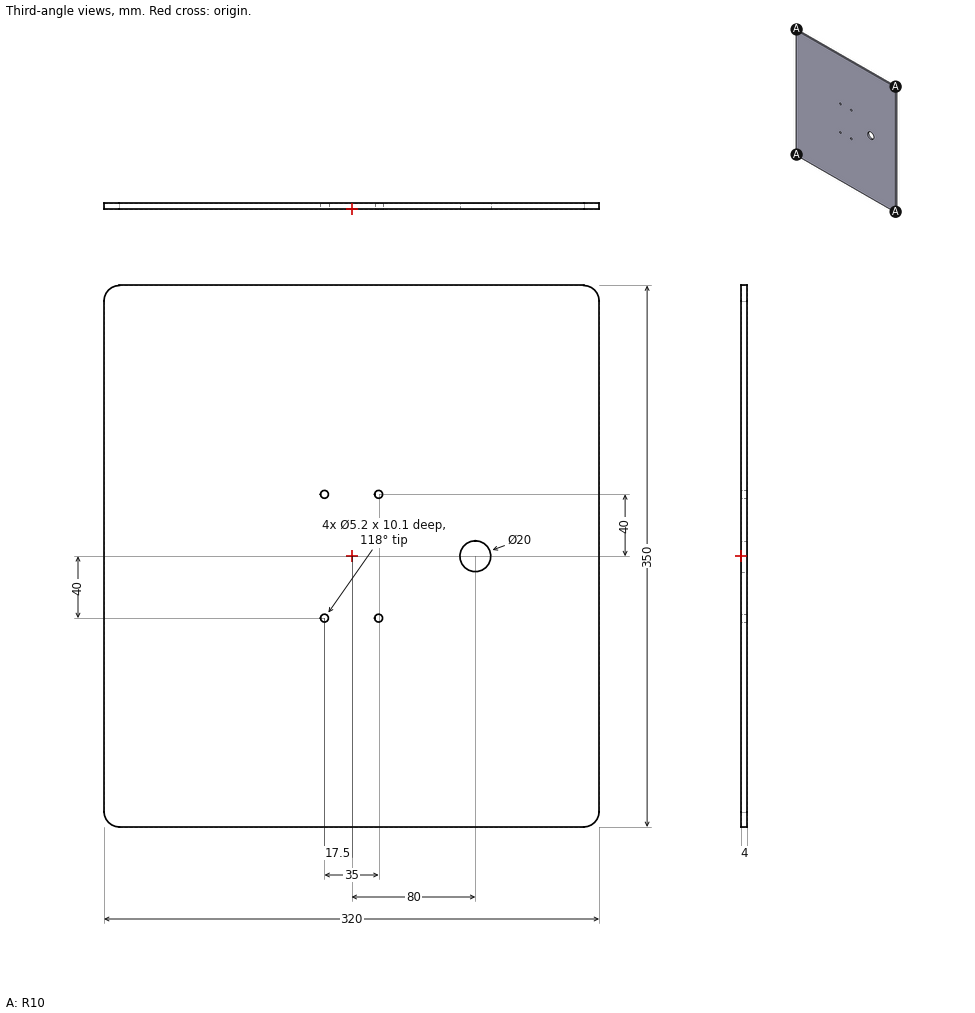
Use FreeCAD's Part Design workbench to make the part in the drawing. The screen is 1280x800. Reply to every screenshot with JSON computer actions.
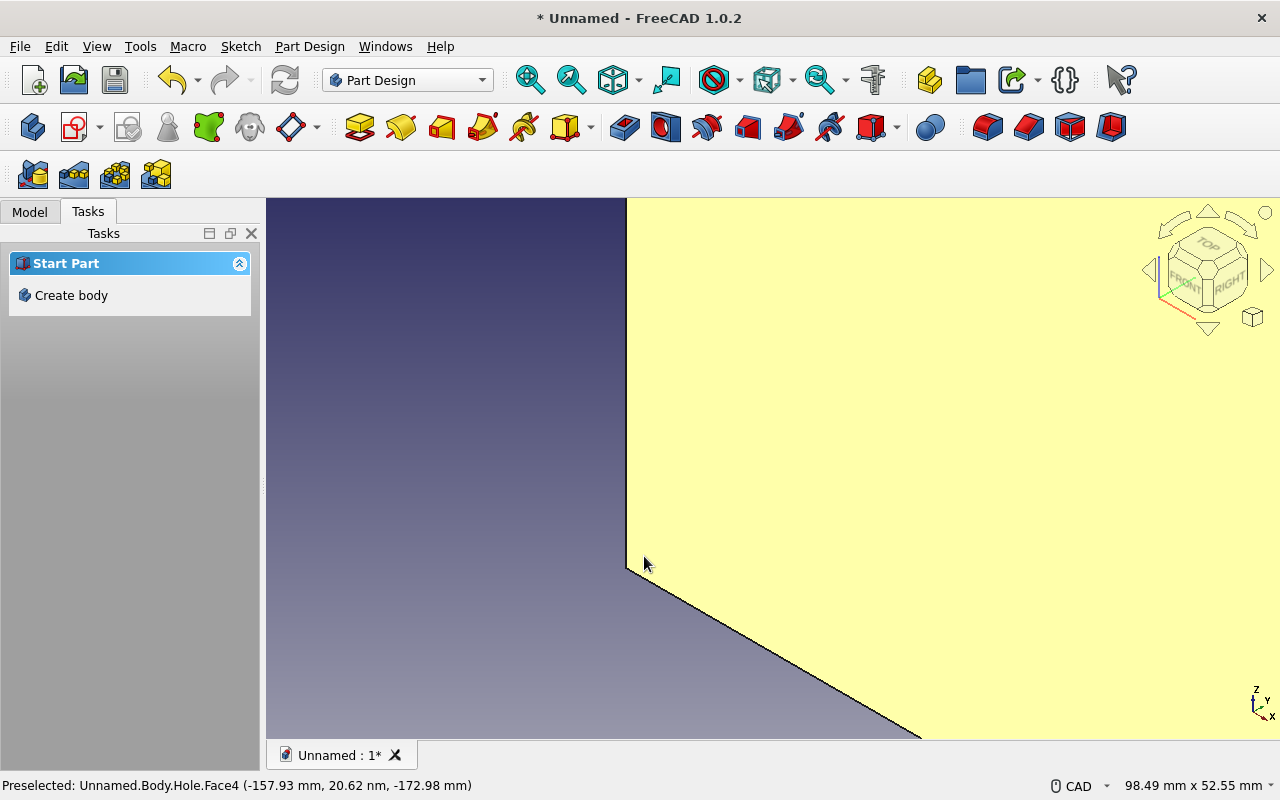
{"action": "key", "text": "v f"}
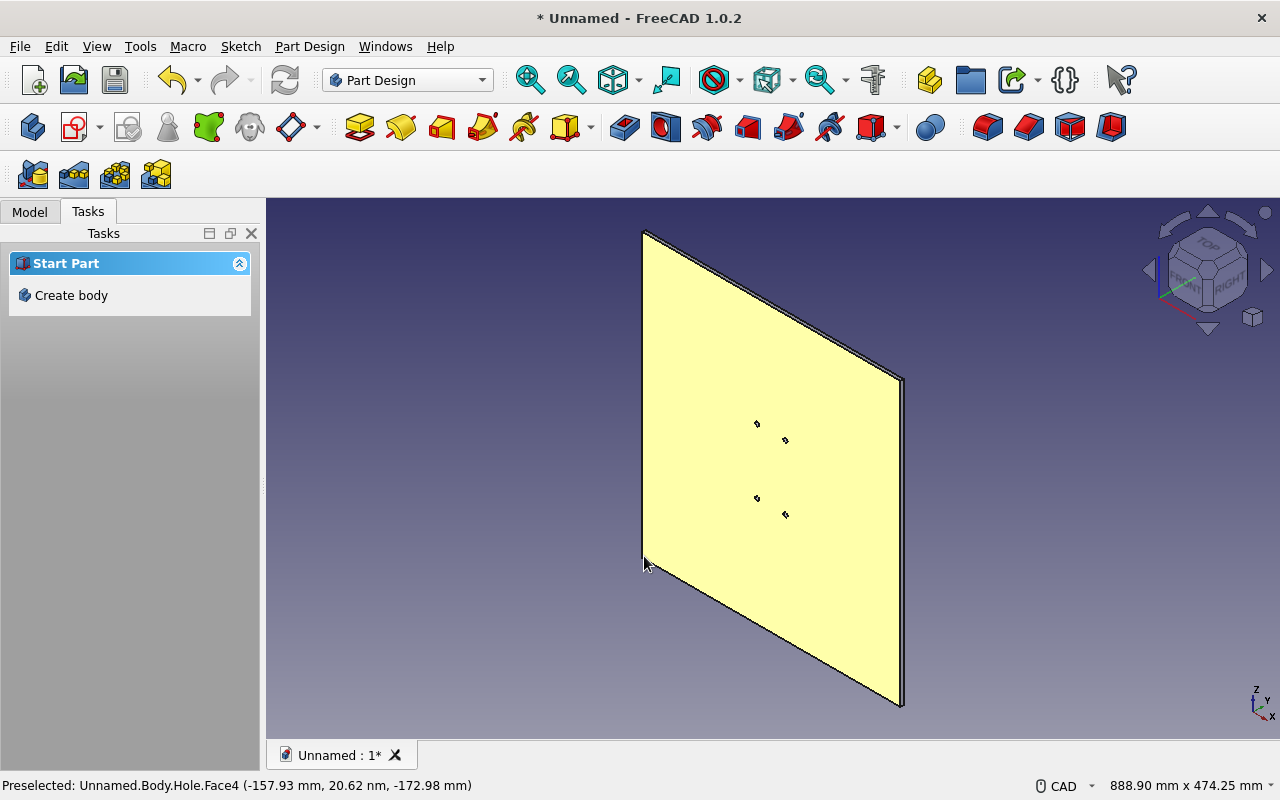
{"action": "key", "text": "2"}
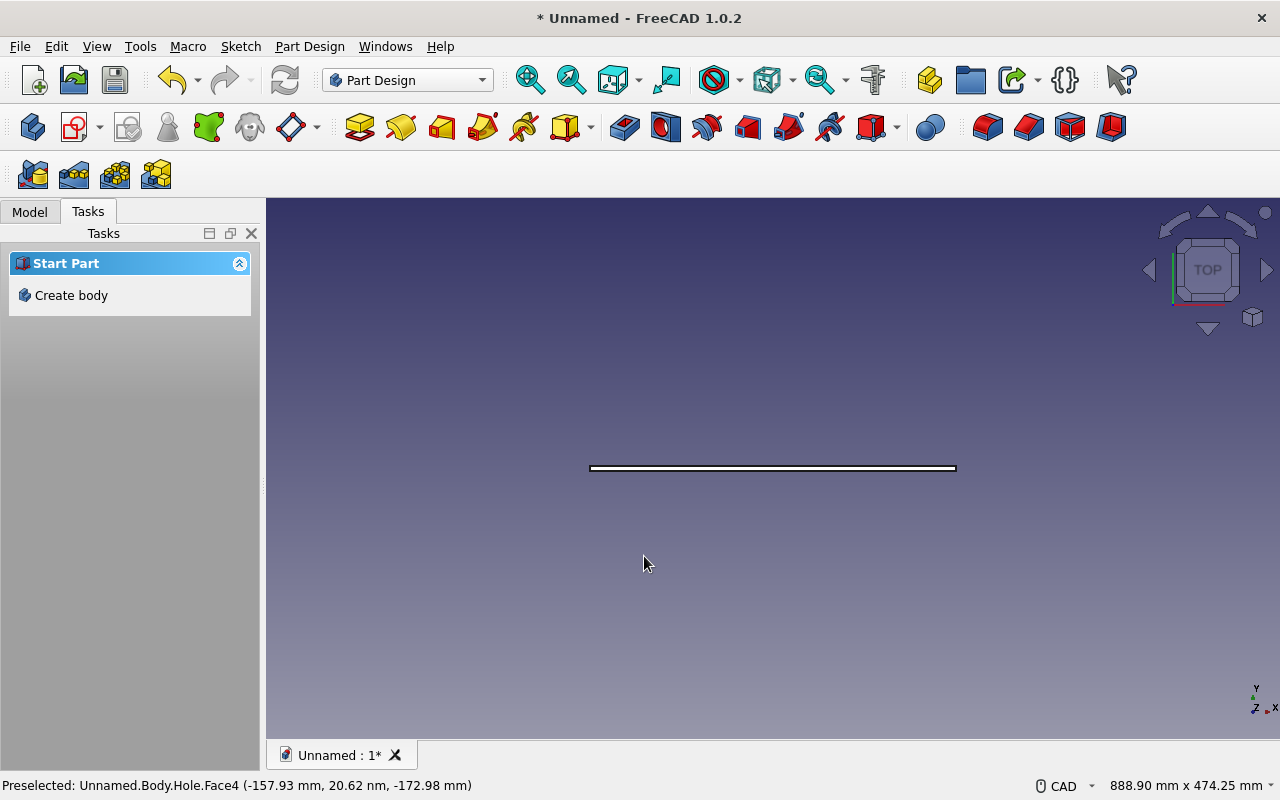
{"action": "left_click", "coordinate": [531, 80]}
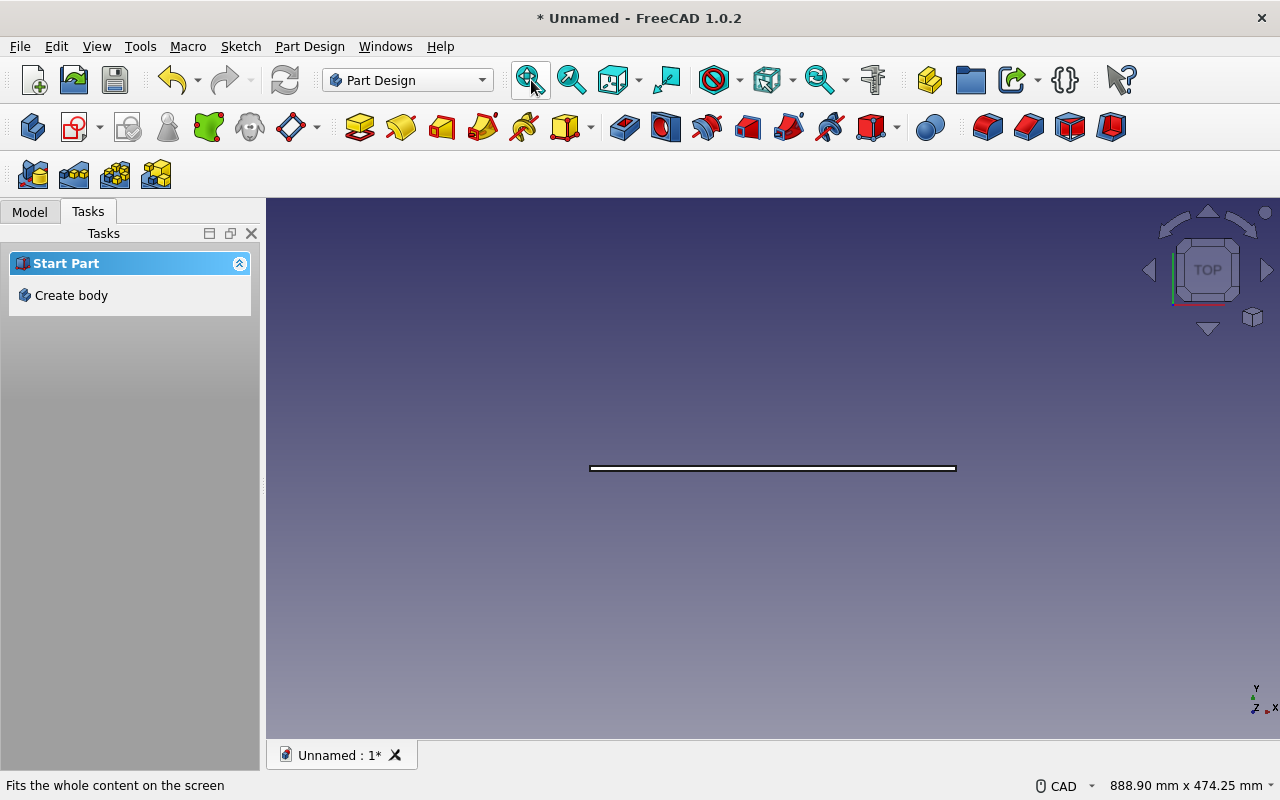
{"action": "scroll", "coordinate": [590, 467], "scroll_direction": "up", "scroll_amount": 11}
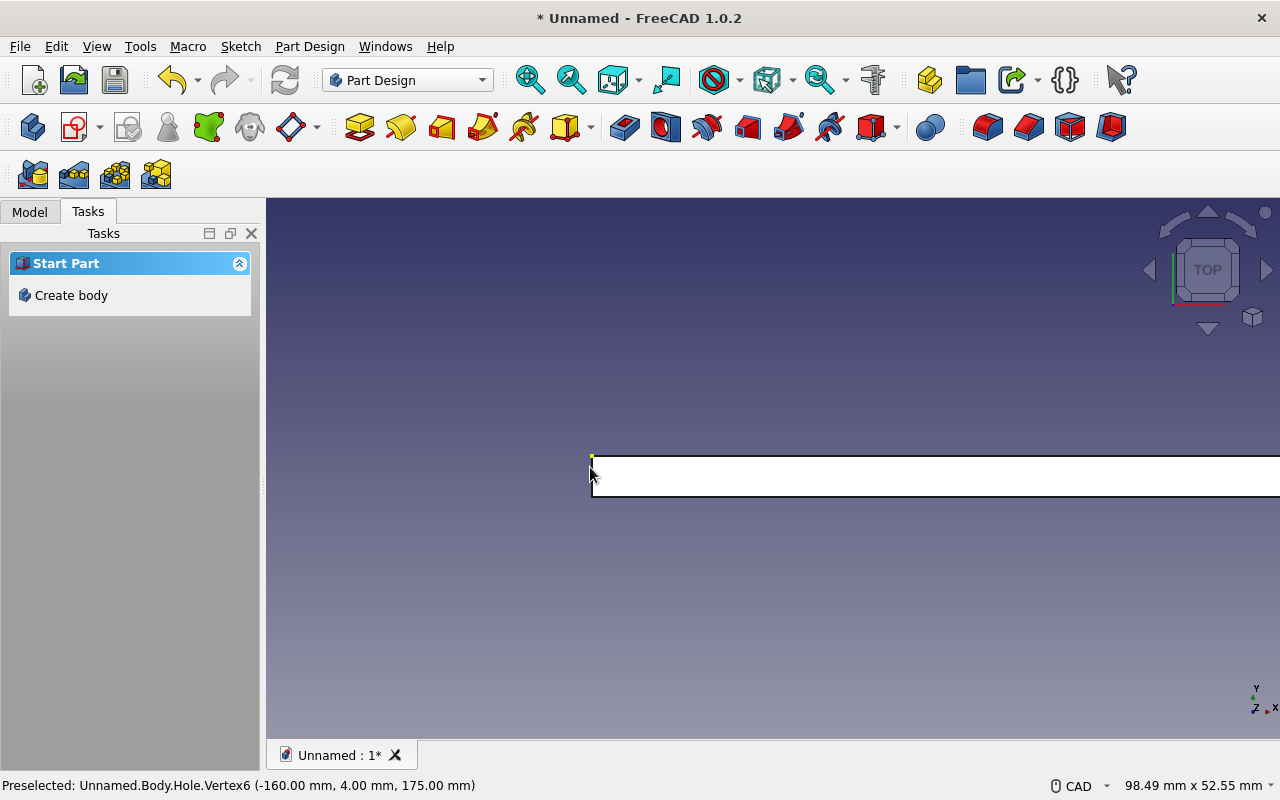
{"action": "left_click", "coordinate": [592, 476]}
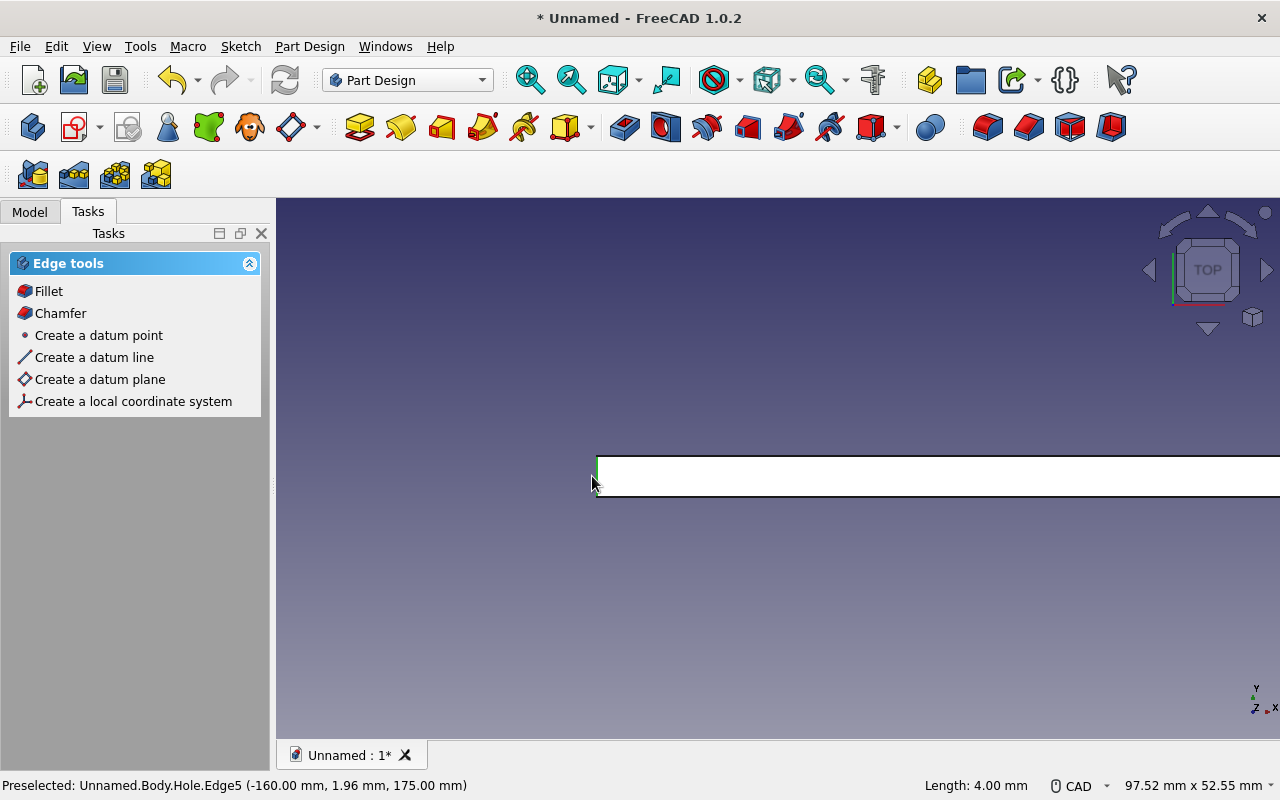
{"action": "key", "text": "v f"}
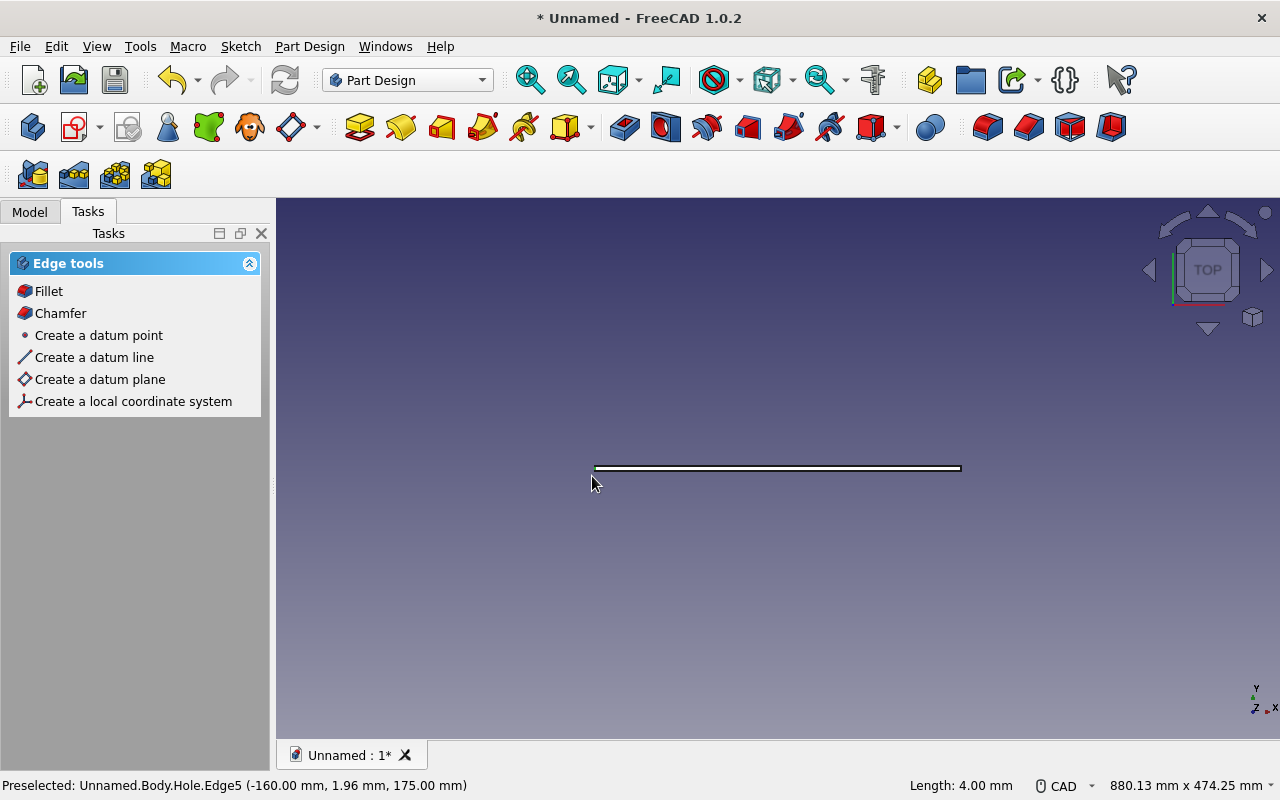
{"action": "key", "text": "1"}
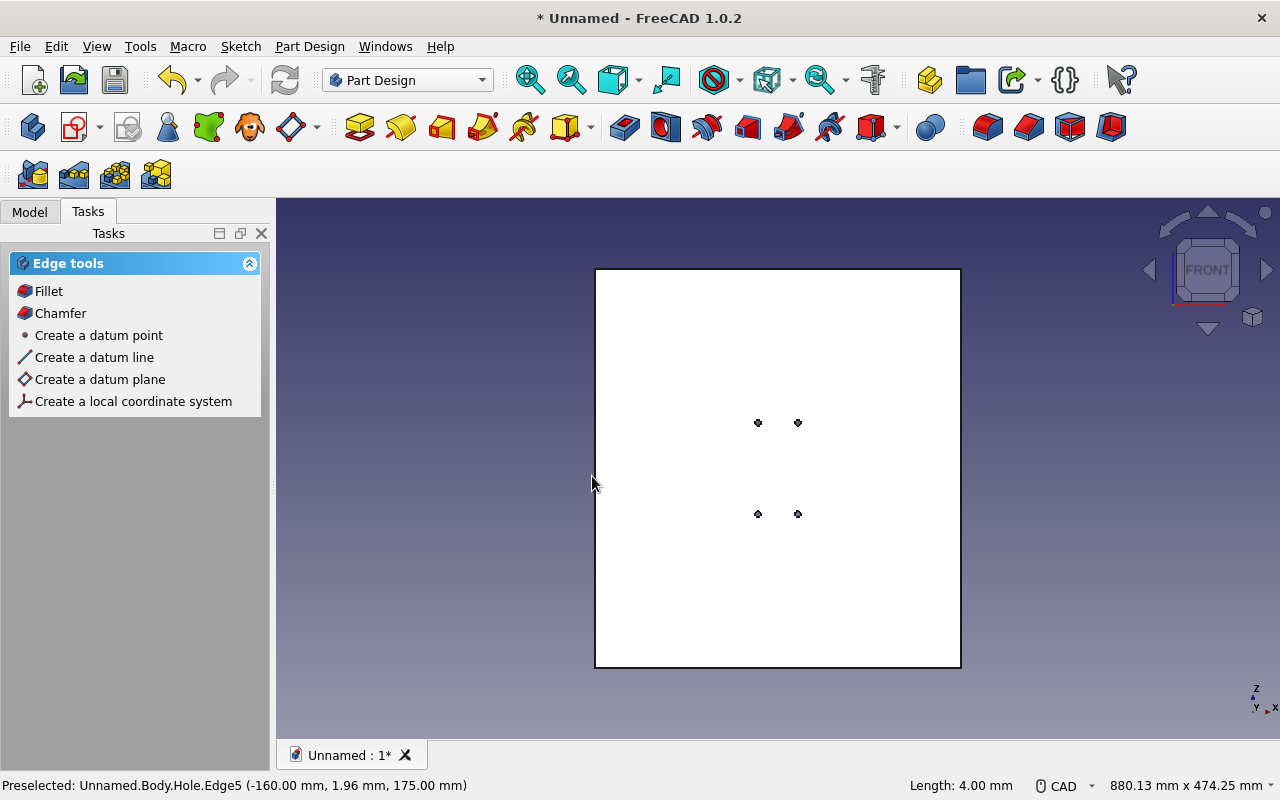
{"action": "scroll", "coordinate": [595, 667], "scroll_direction": "up", "scroll_amount": 11}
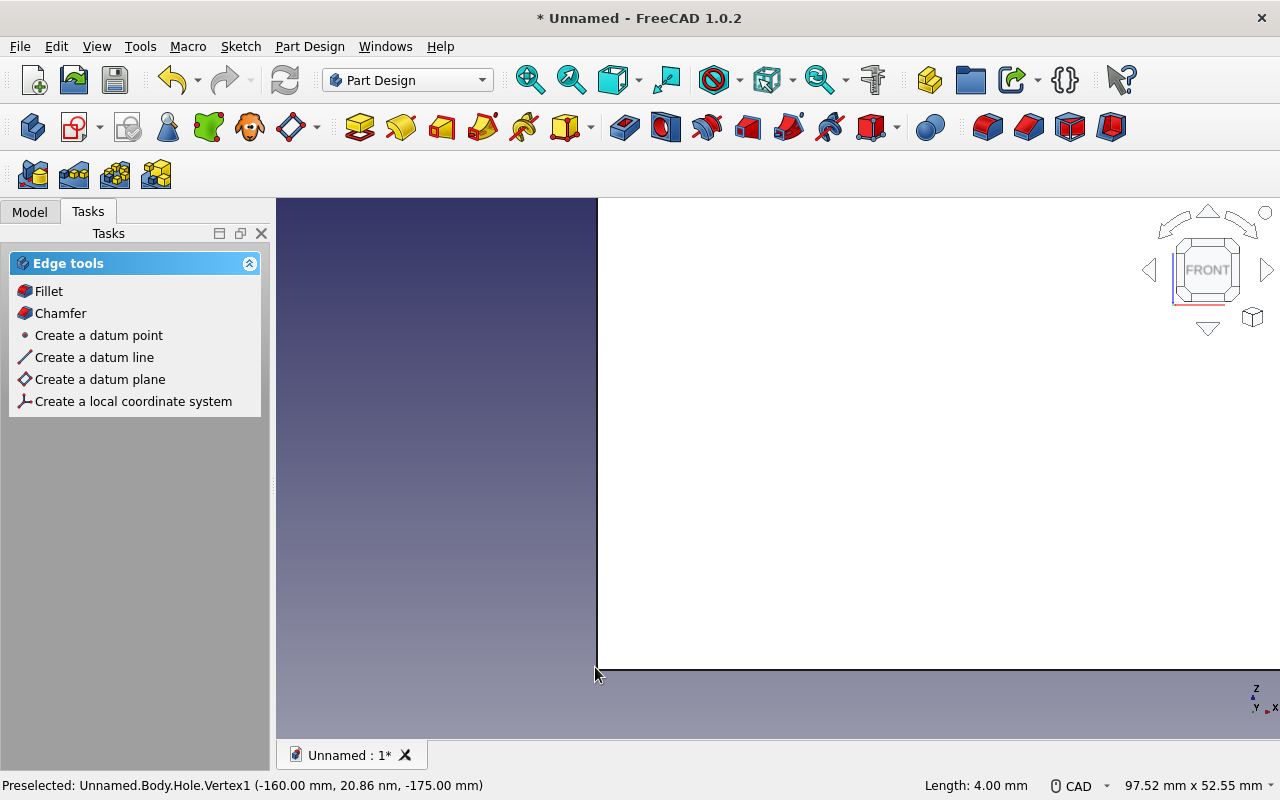
{"action": "left_click", "coordinate": [531, 80]}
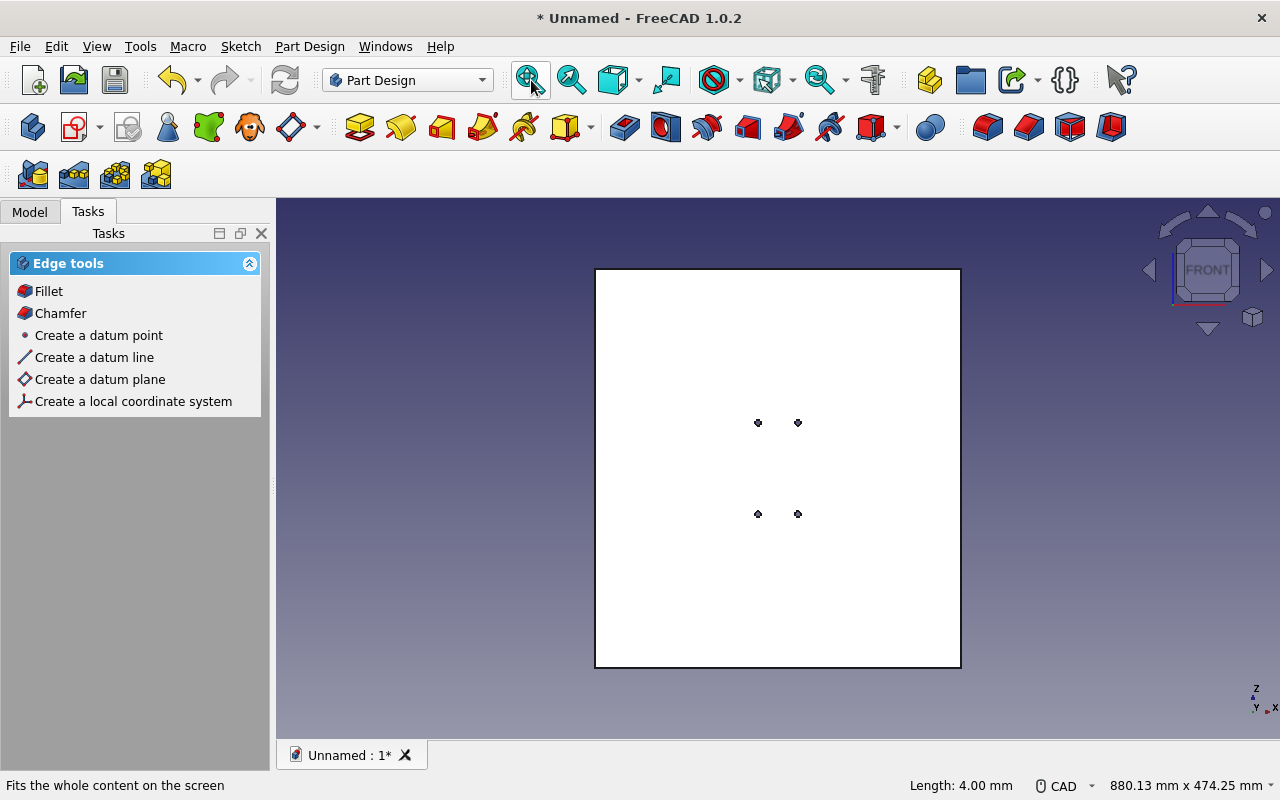
{"action": "key", "text": "3"}